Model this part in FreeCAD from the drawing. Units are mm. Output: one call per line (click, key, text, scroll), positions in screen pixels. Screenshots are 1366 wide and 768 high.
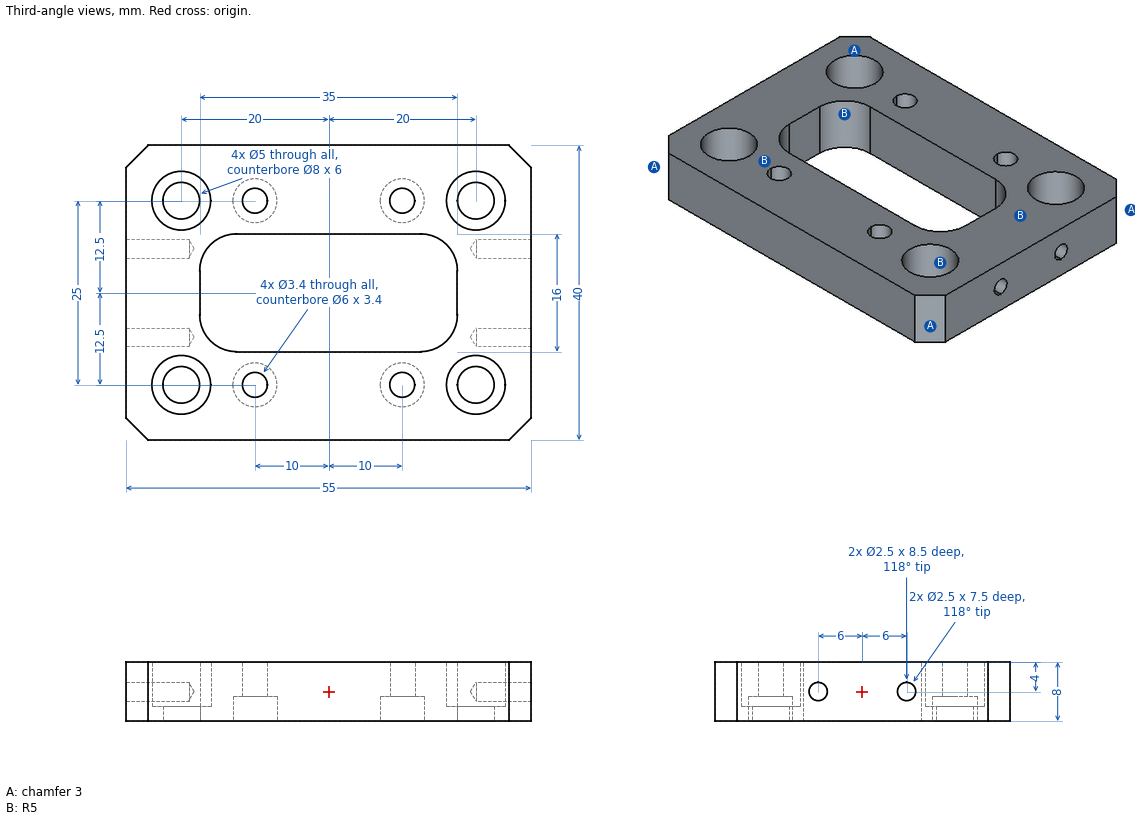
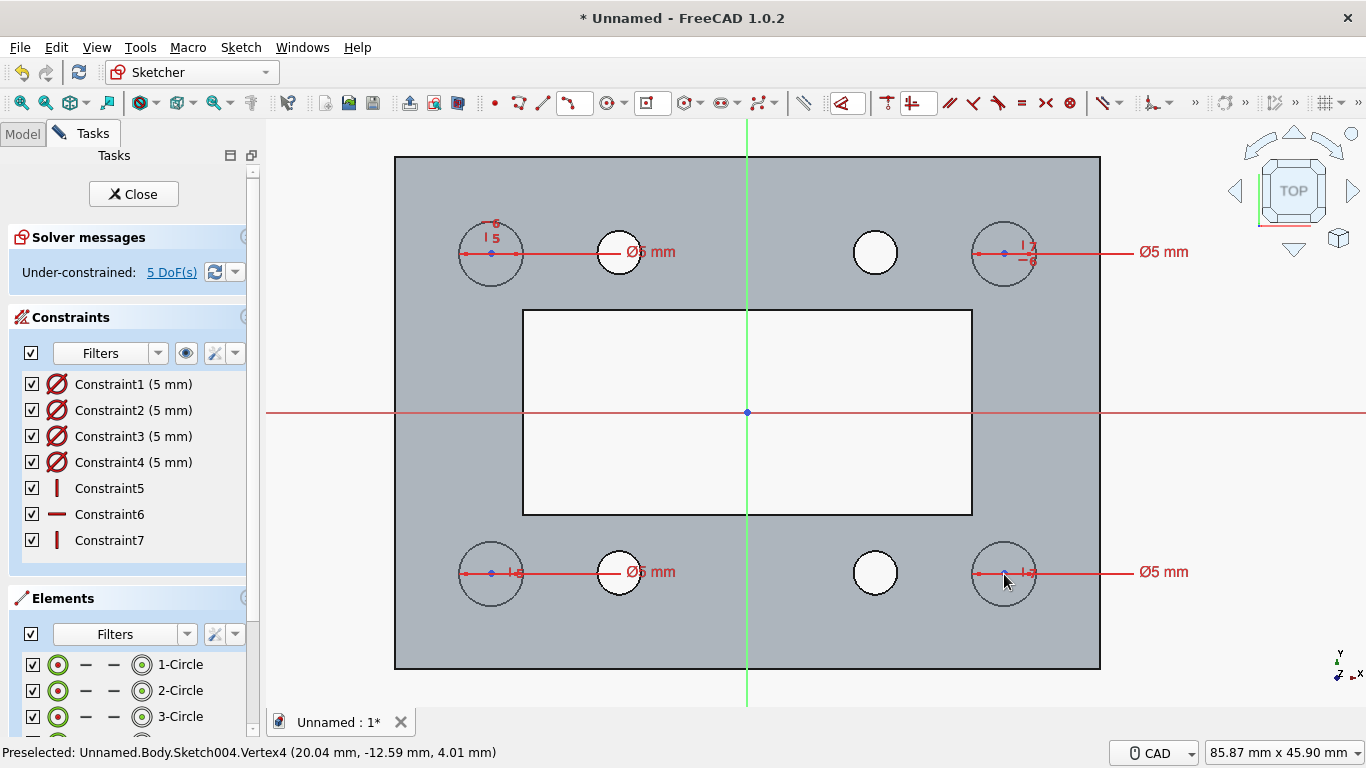
click(491, 574)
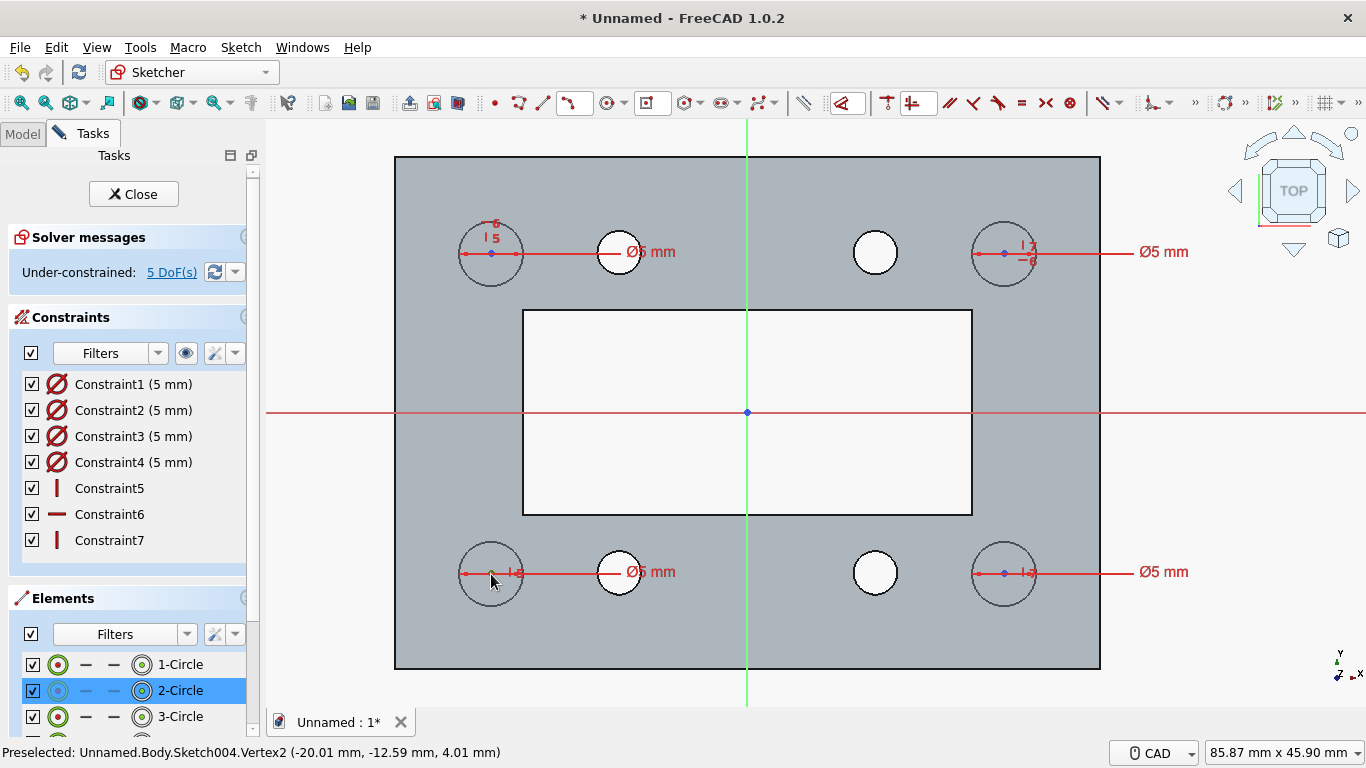
click(1004, 574)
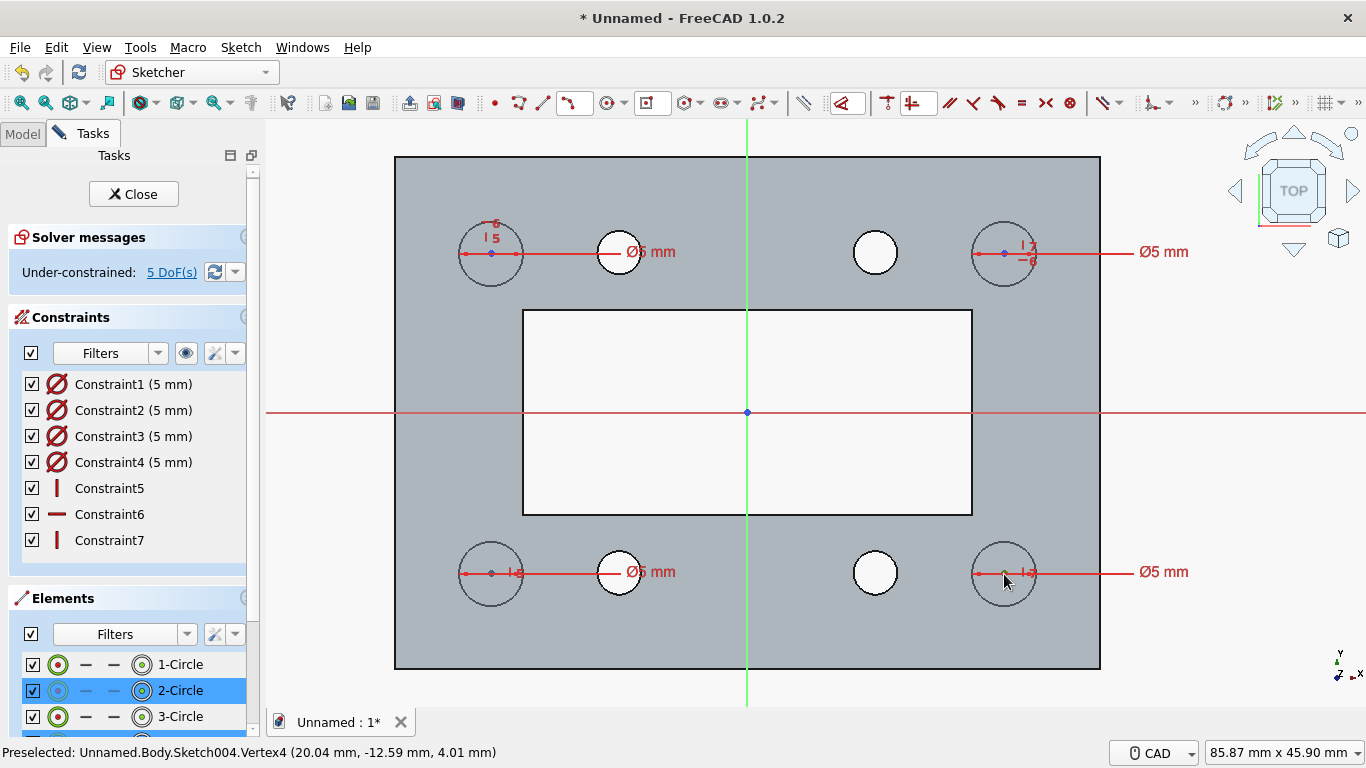
click(932, 104)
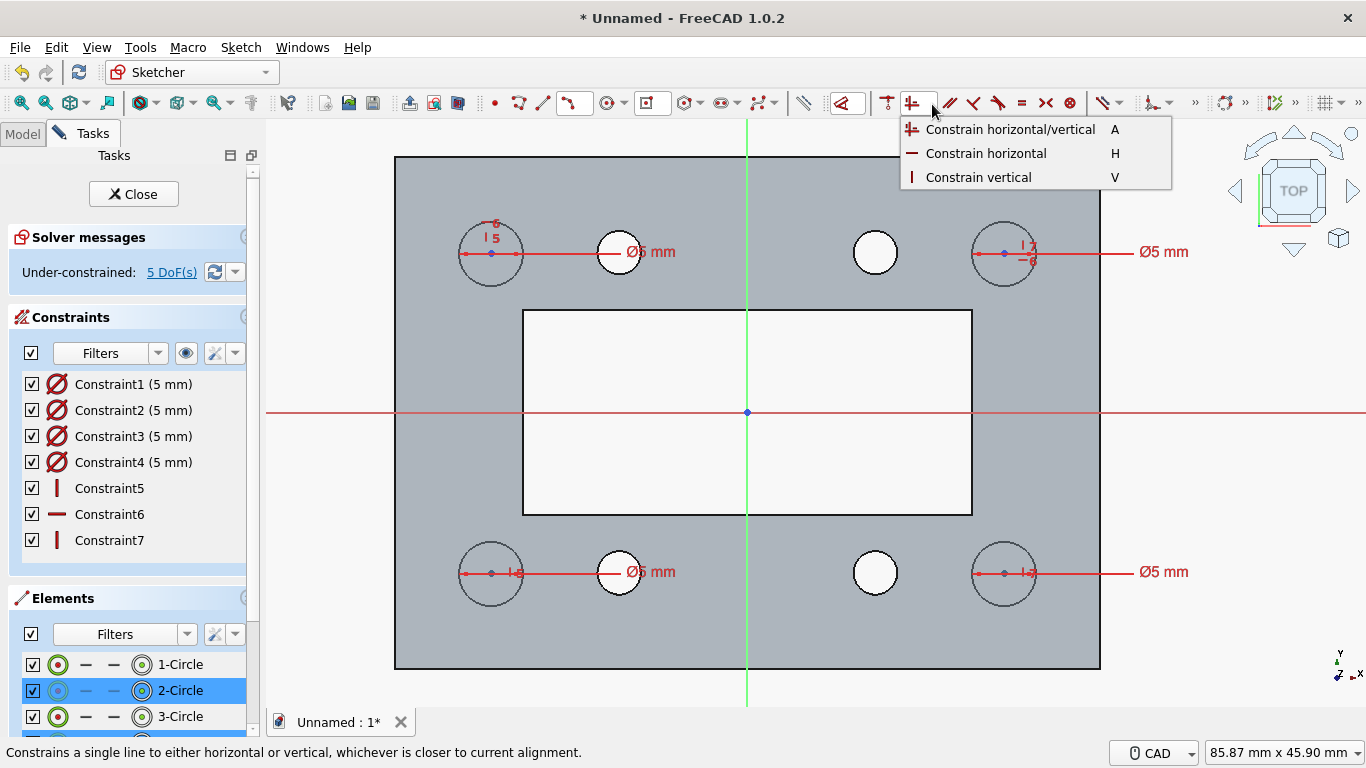
click(1036, 153)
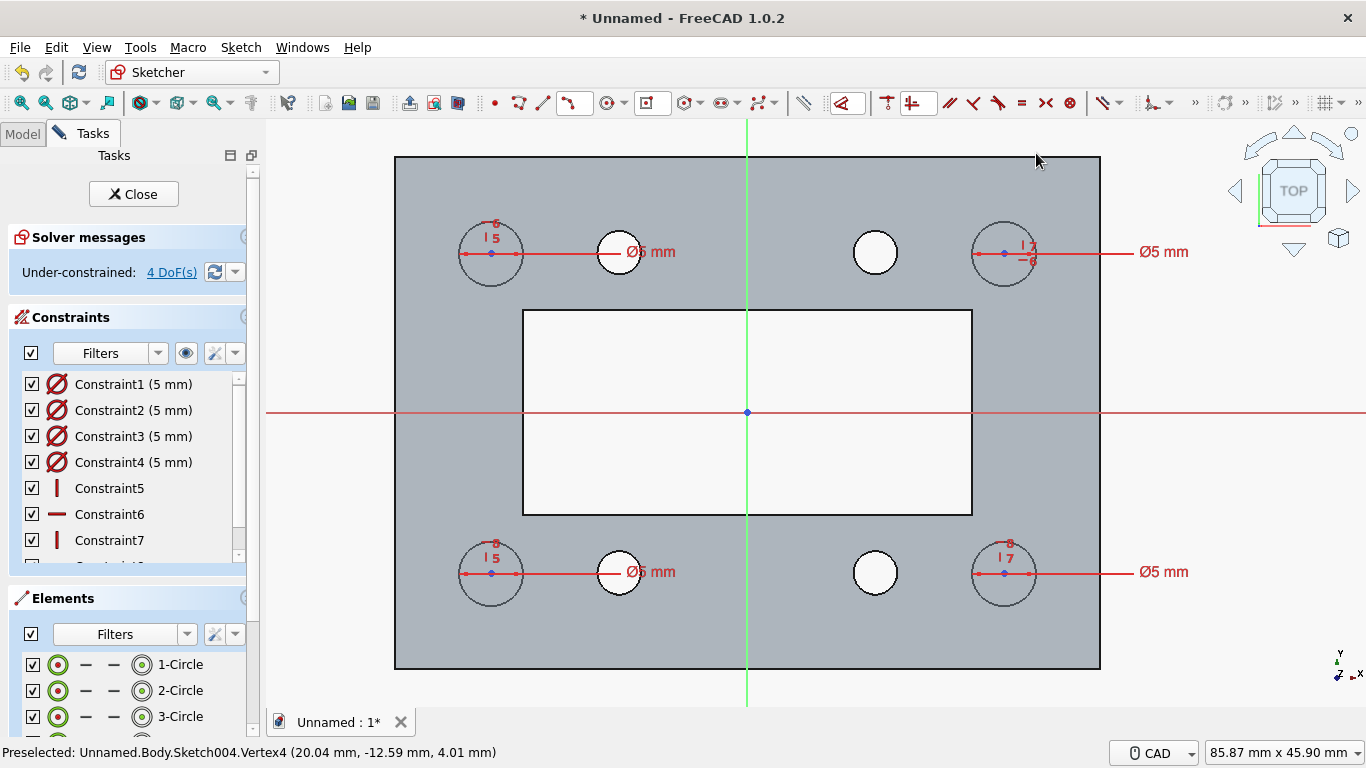
click(491, 254)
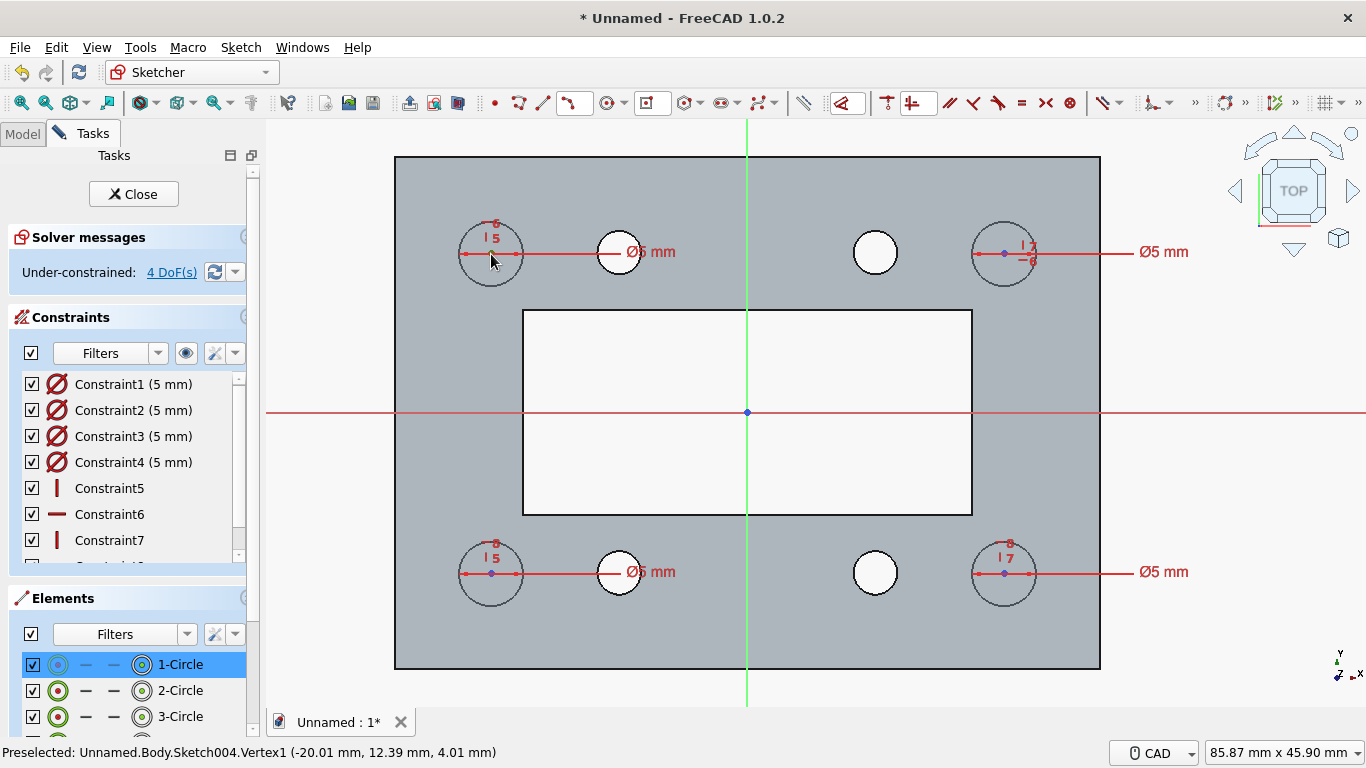
click(860, 104)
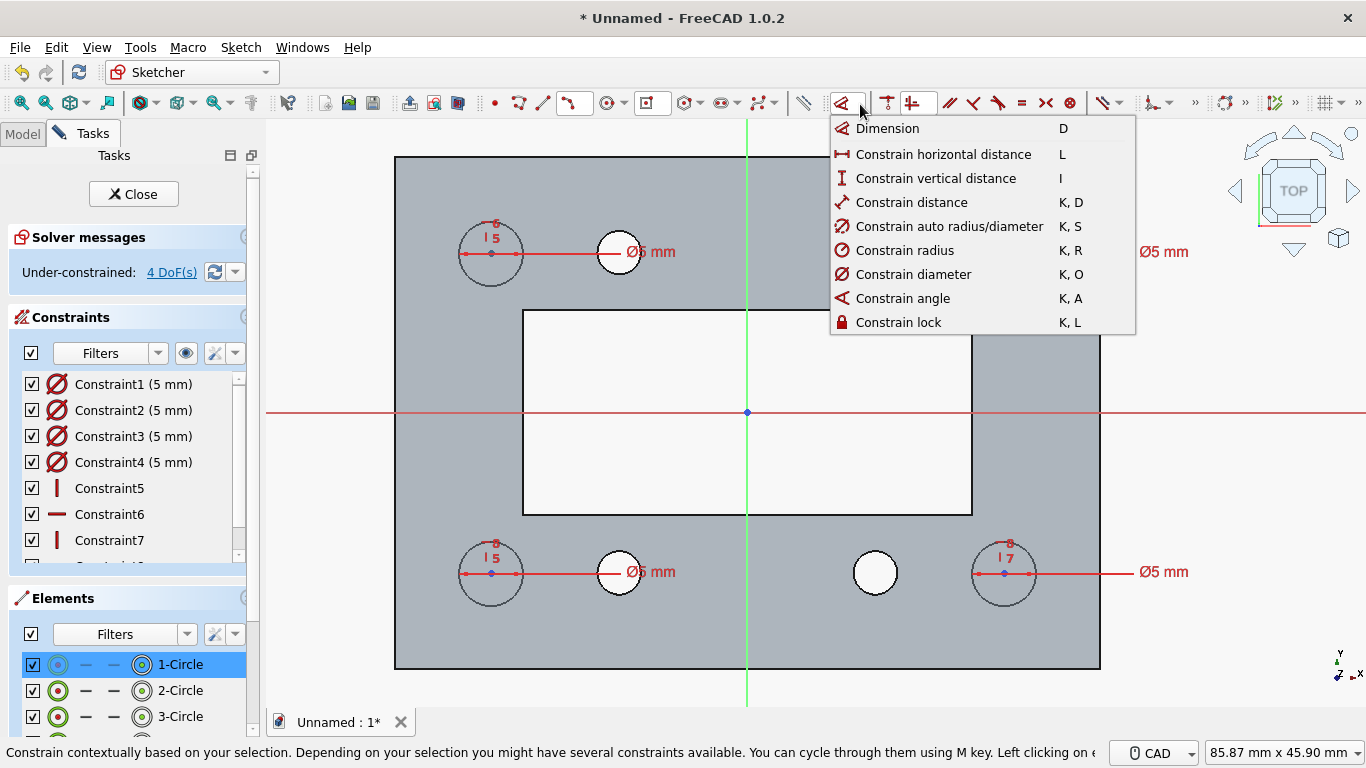
click(983, 154)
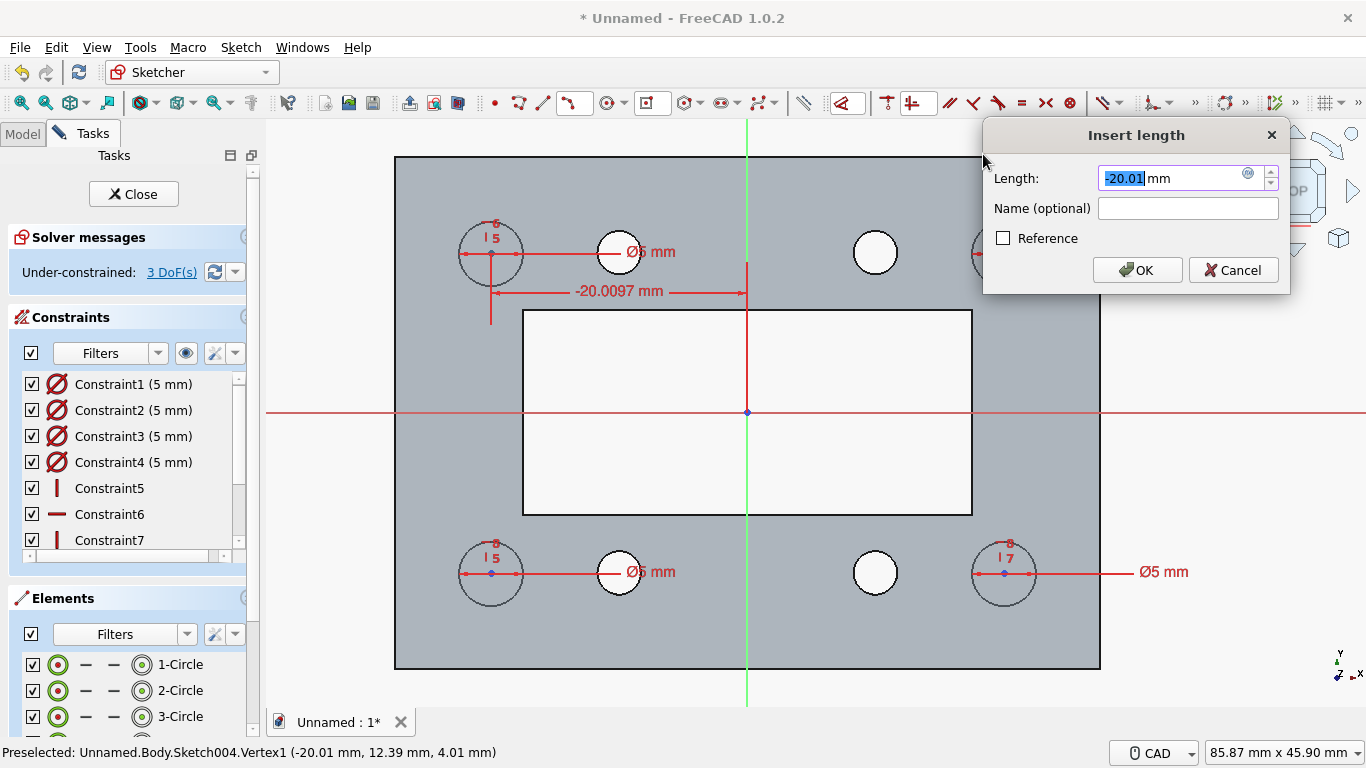
text(-20)
key(Return)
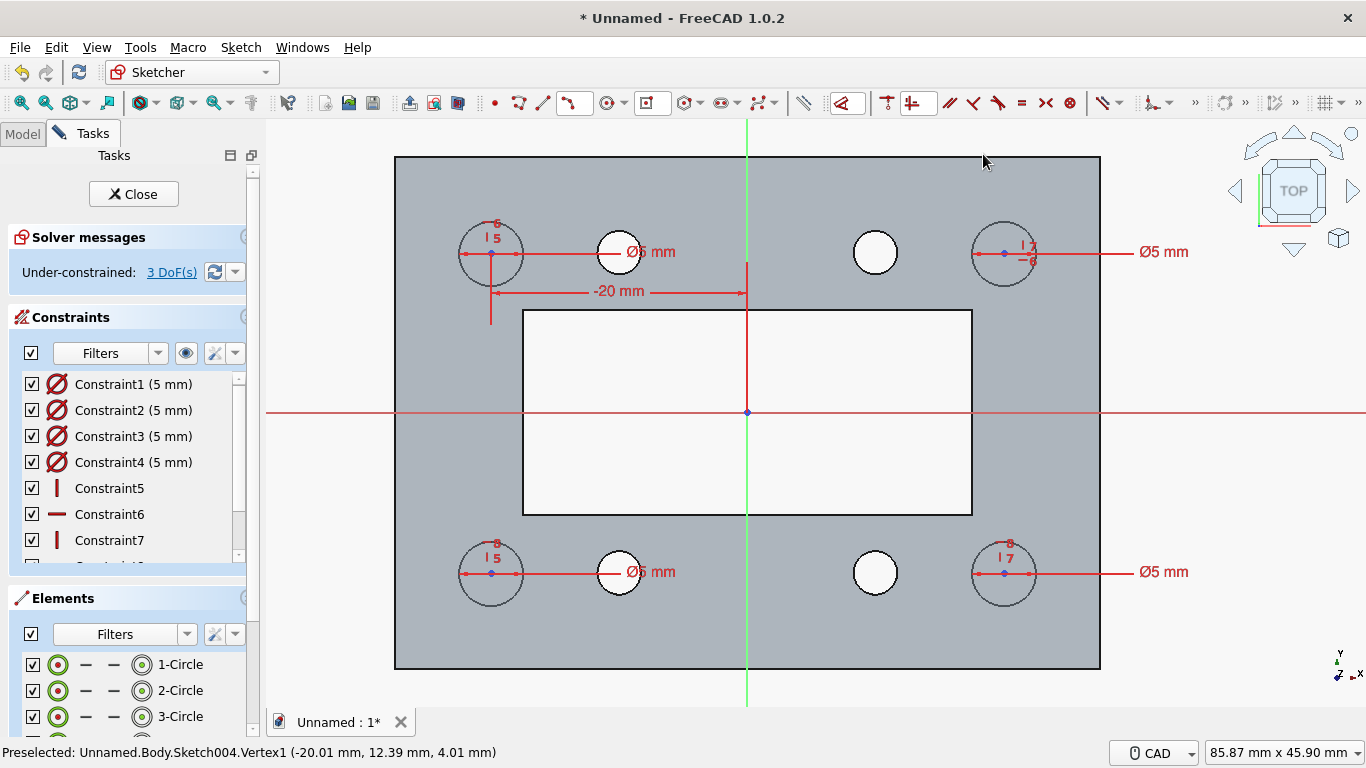
click(1004, 254)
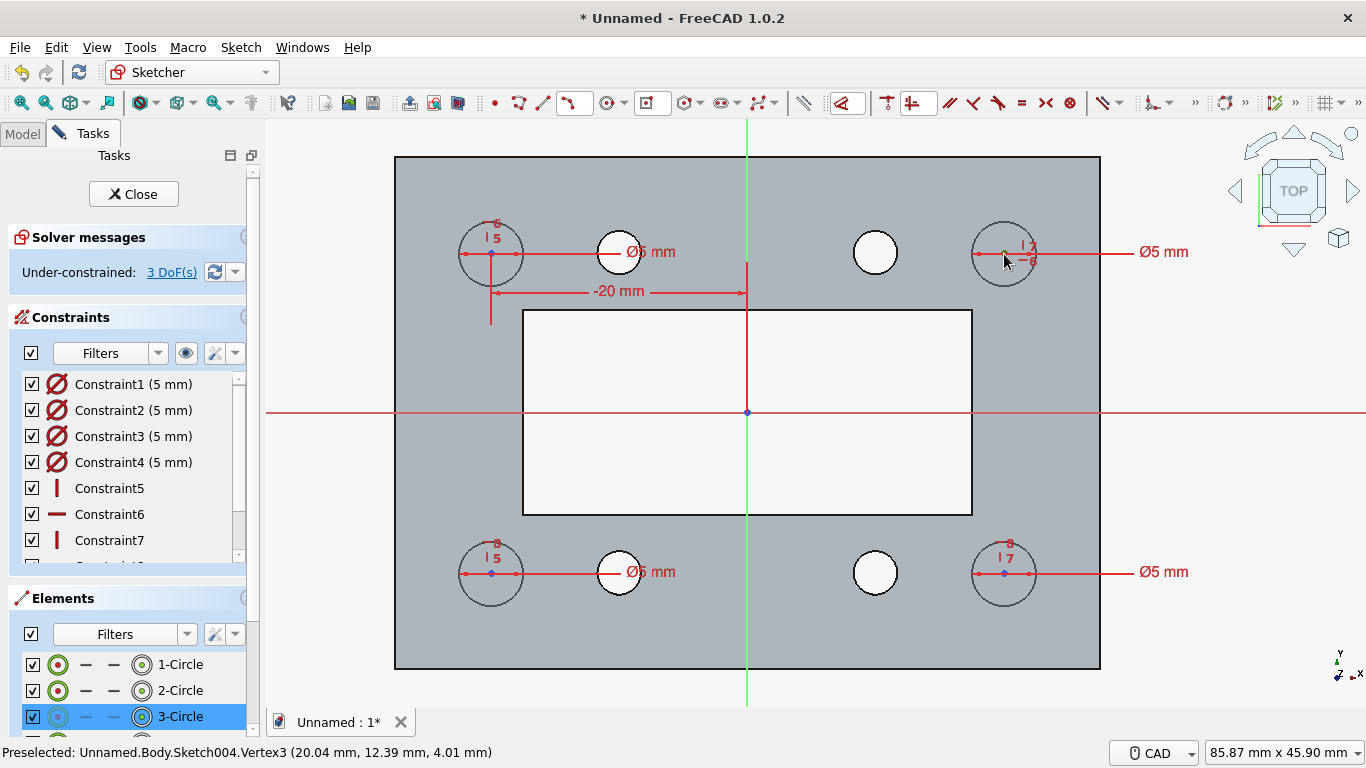
key(l)